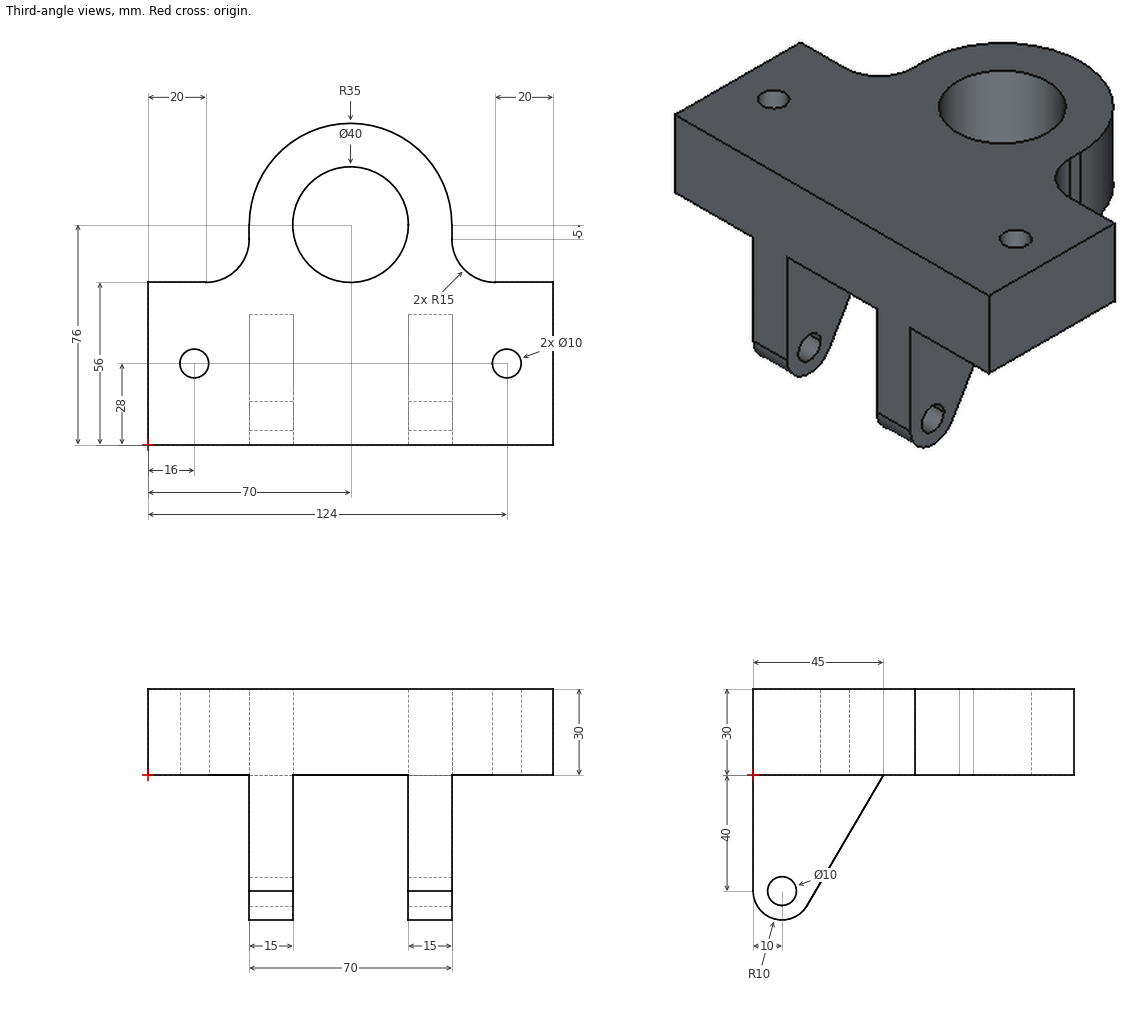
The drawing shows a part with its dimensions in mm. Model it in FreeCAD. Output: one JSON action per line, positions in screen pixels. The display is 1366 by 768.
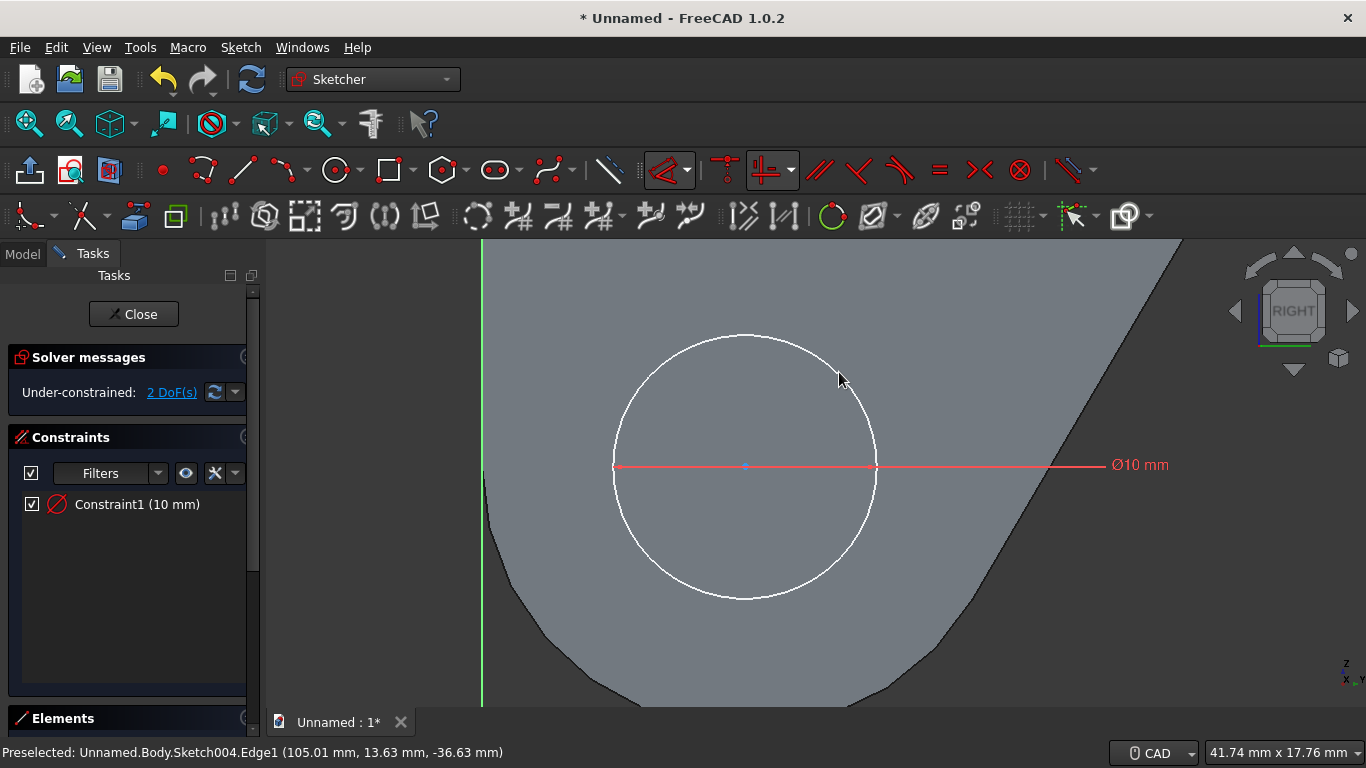
{"action": "left_click", "coordinate": [745, 467]}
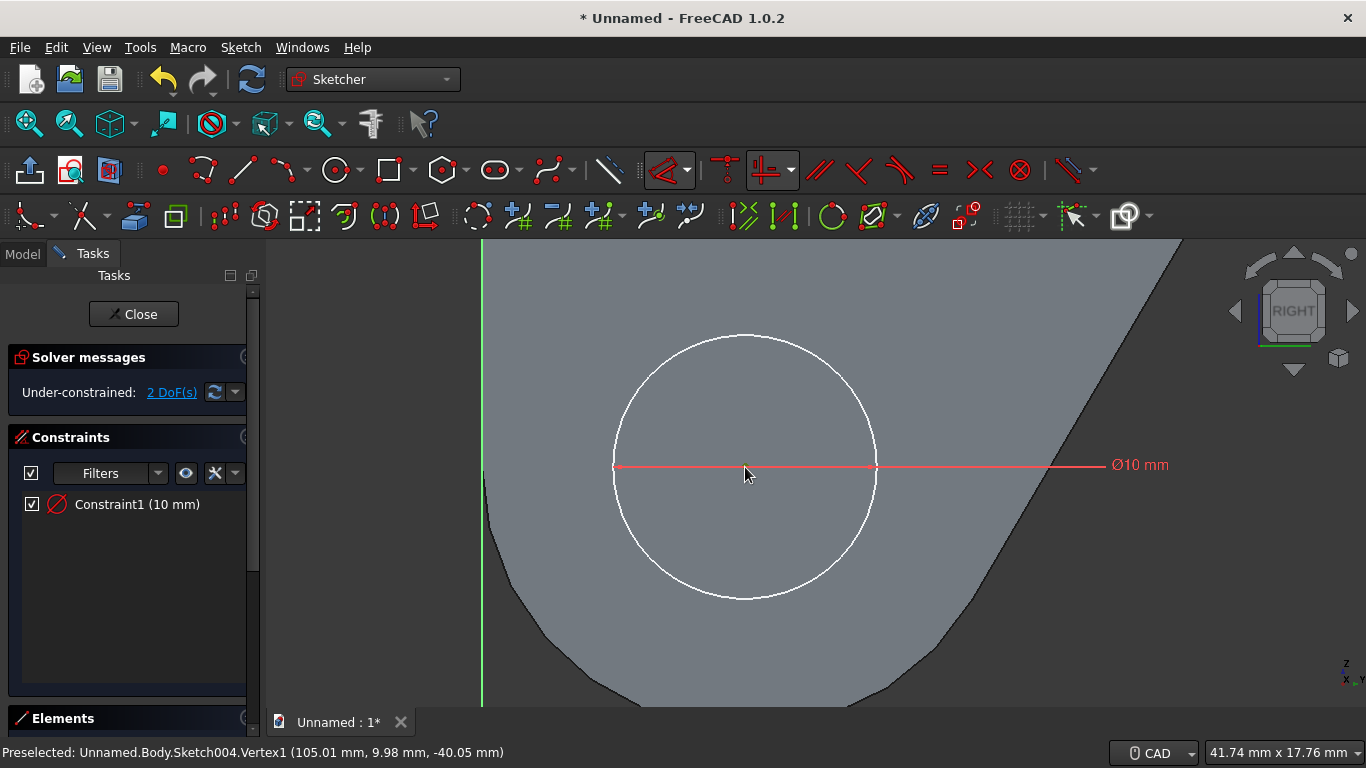
{"action": "left_click", "coordinate": [690, 170]}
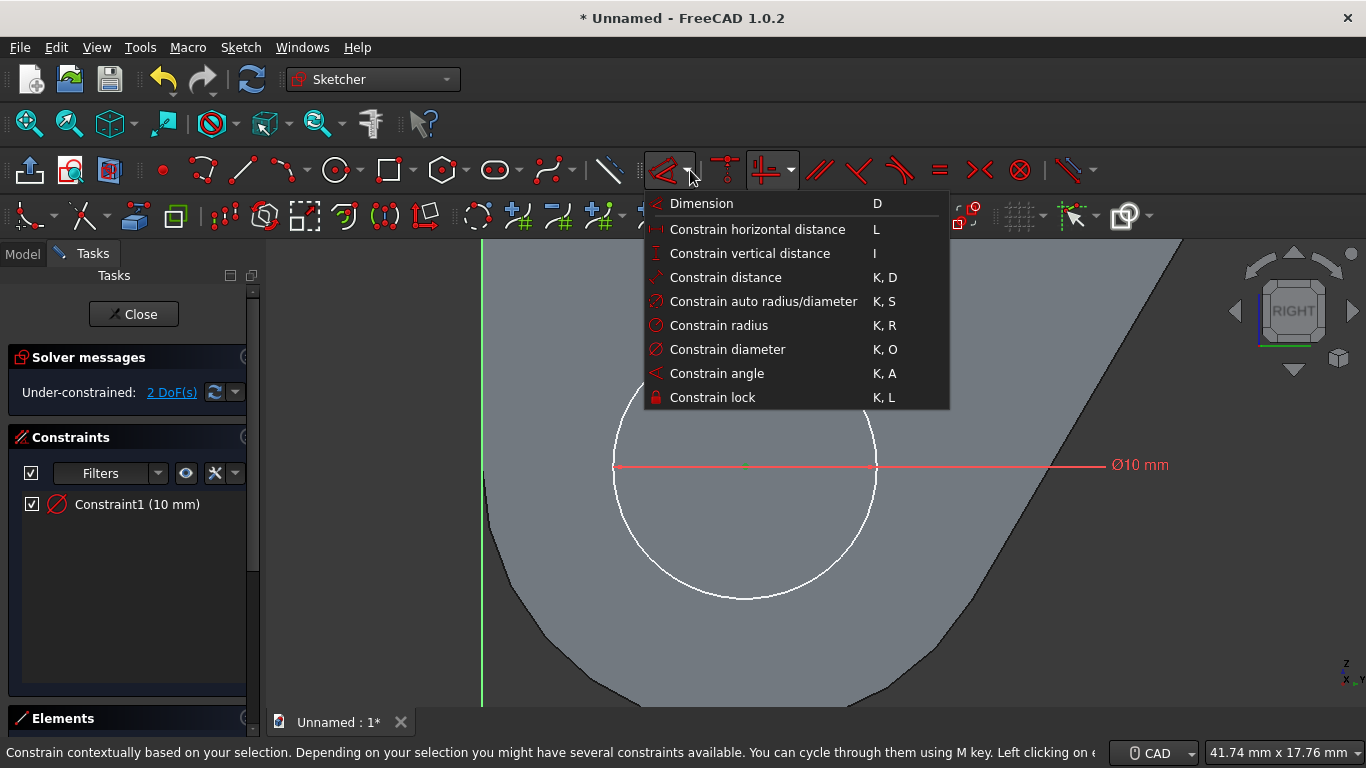
{"action": "left_click", "coordinate": [797, 229]}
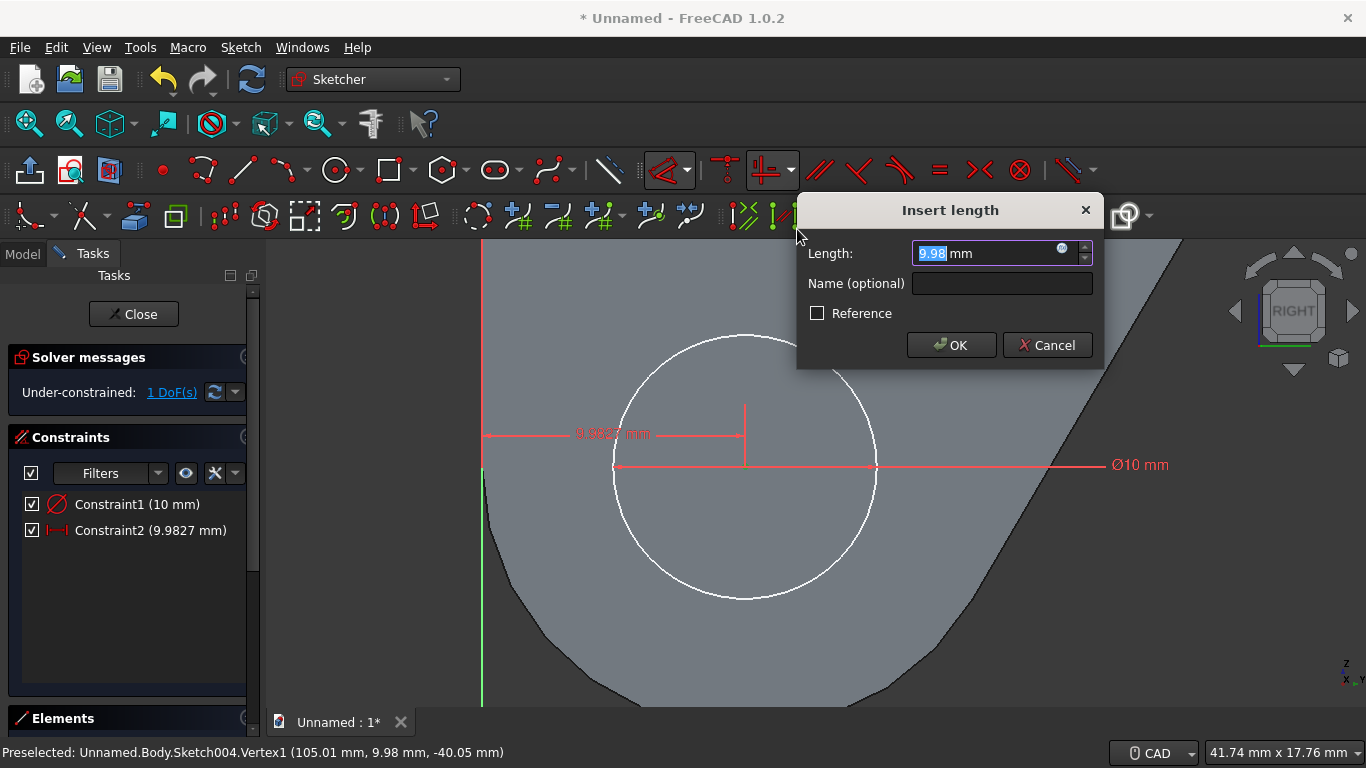
{"action": "type", "text": "10"}
{"action": "key", "text": "Return"}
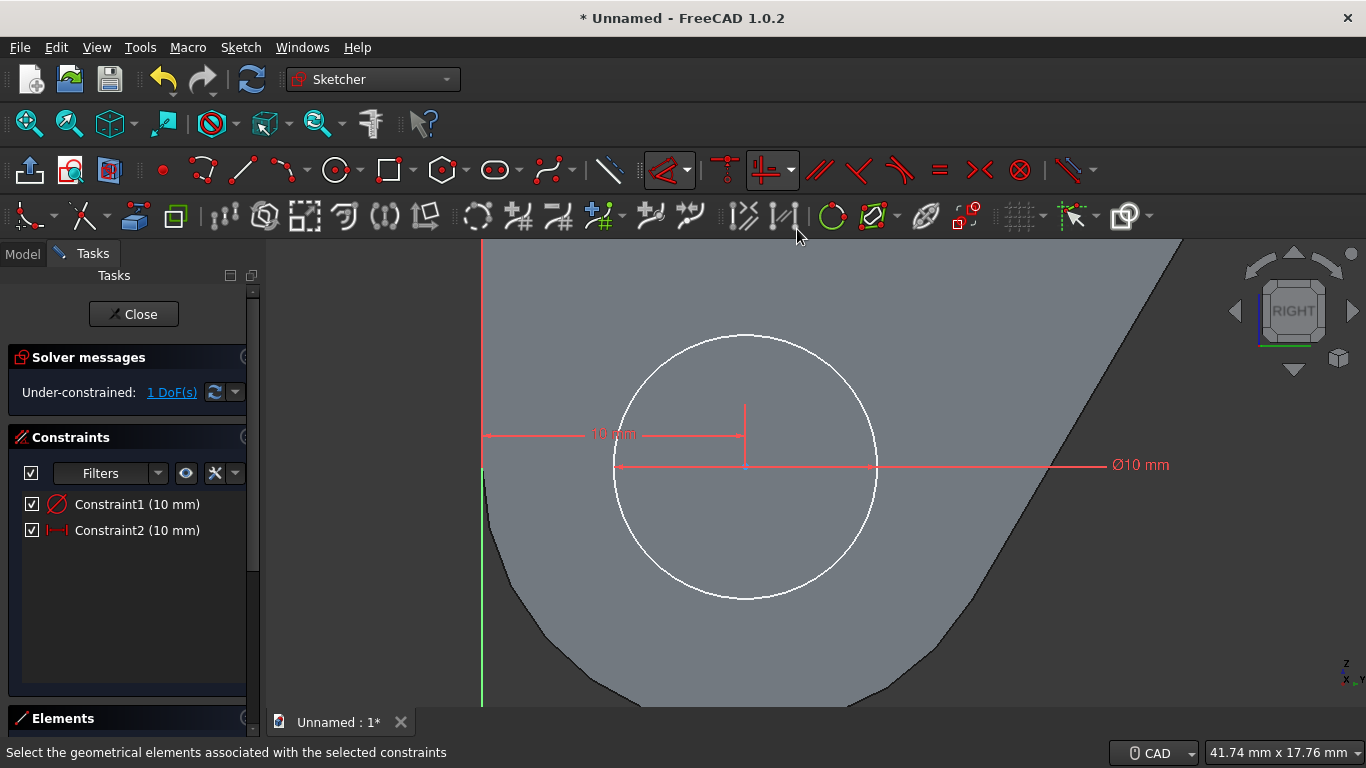
{"action": "left_click", "coordinate": [745, 467]}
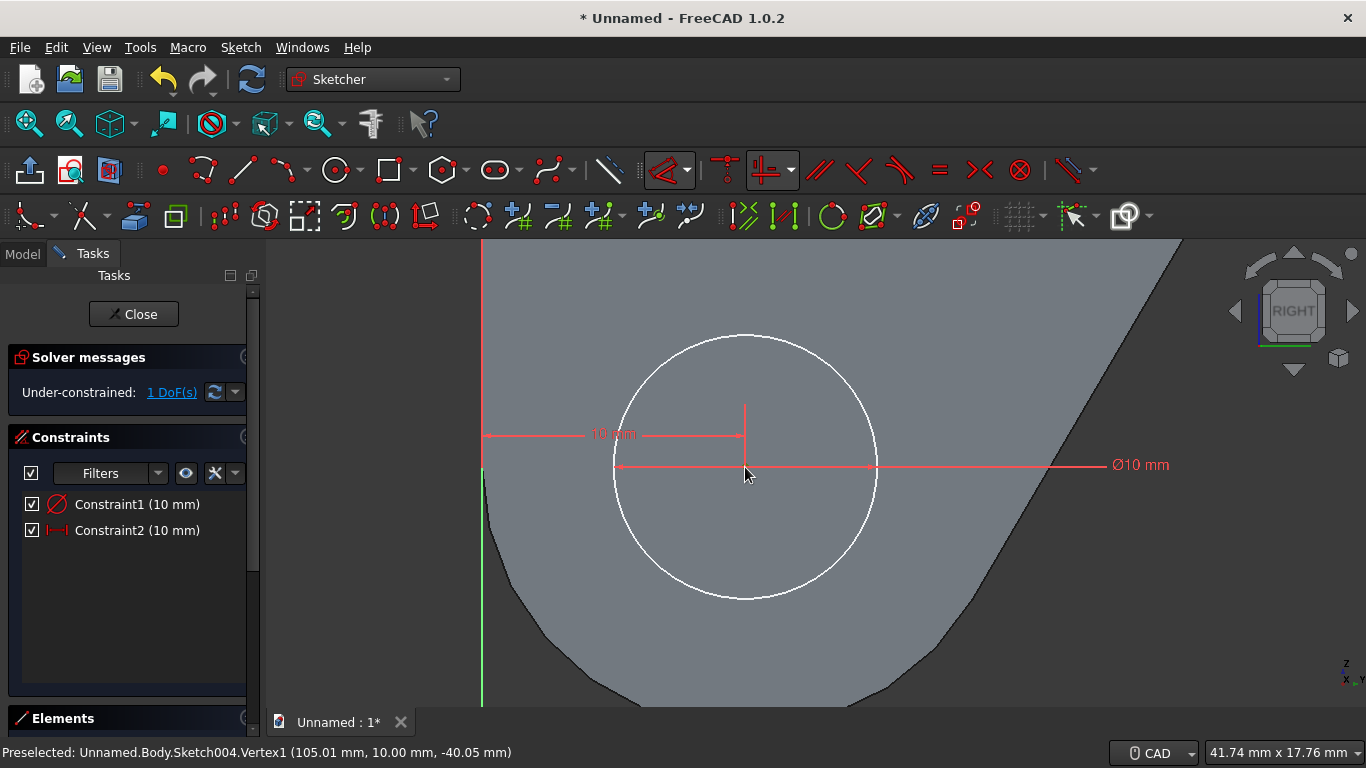
{"action": "key", "text": "i"}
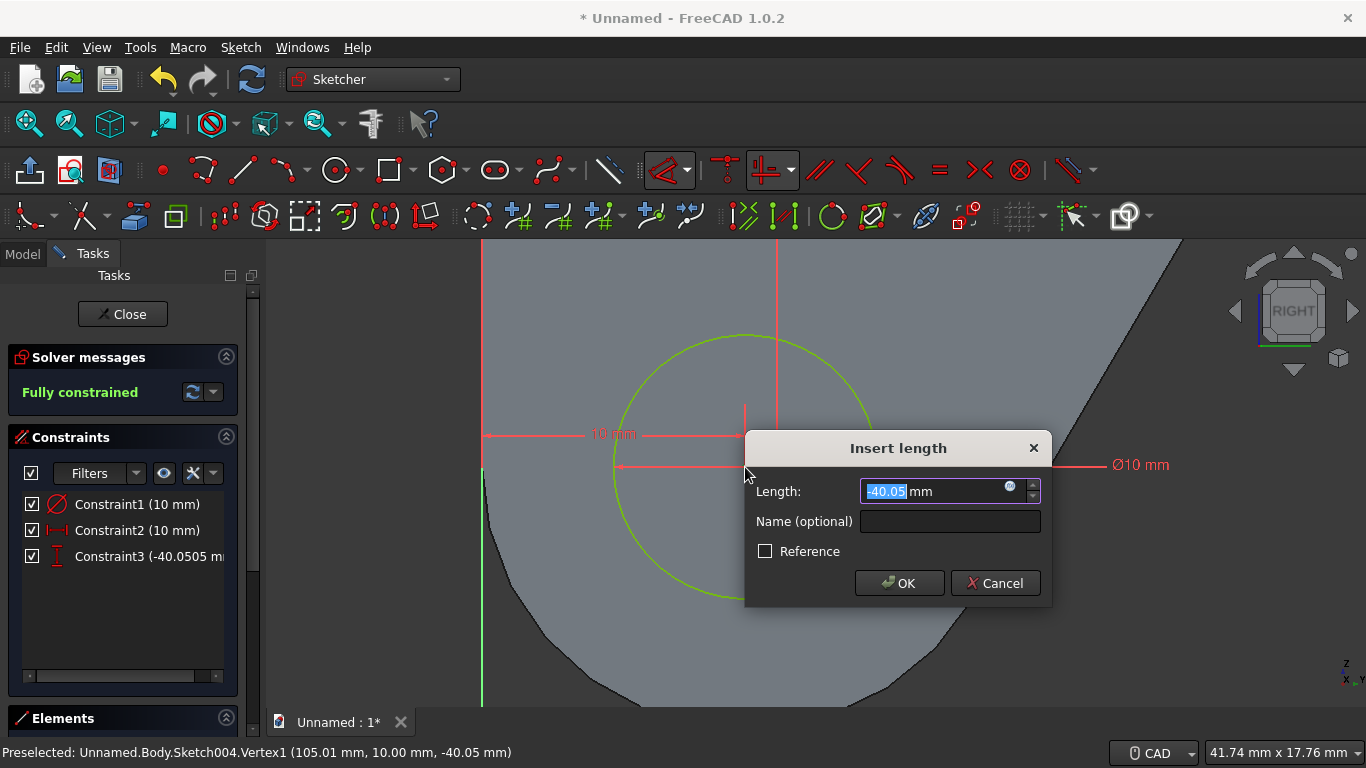
{"action": "type", "text": "-40"}
{"action": "key", "text": "Return"}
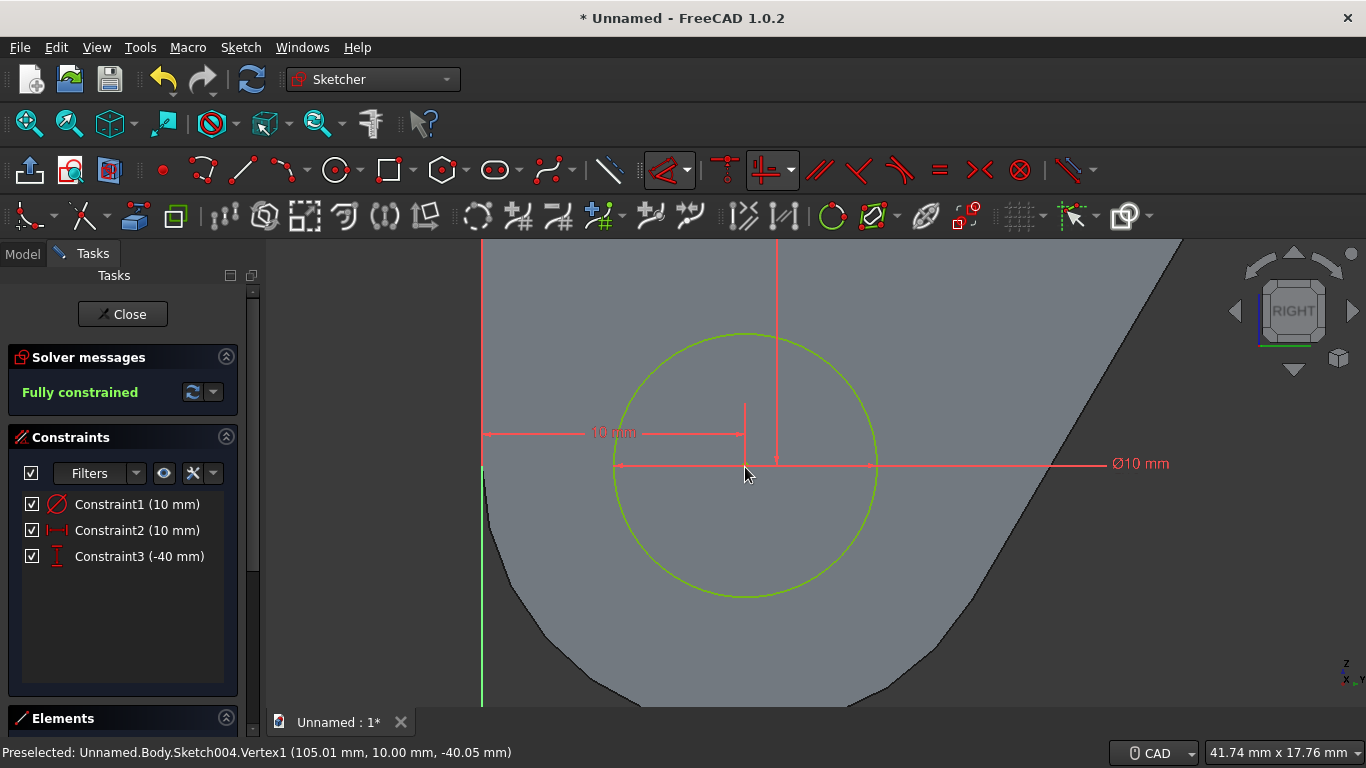
{"action": "left_click", "coordinate": [123, 314]}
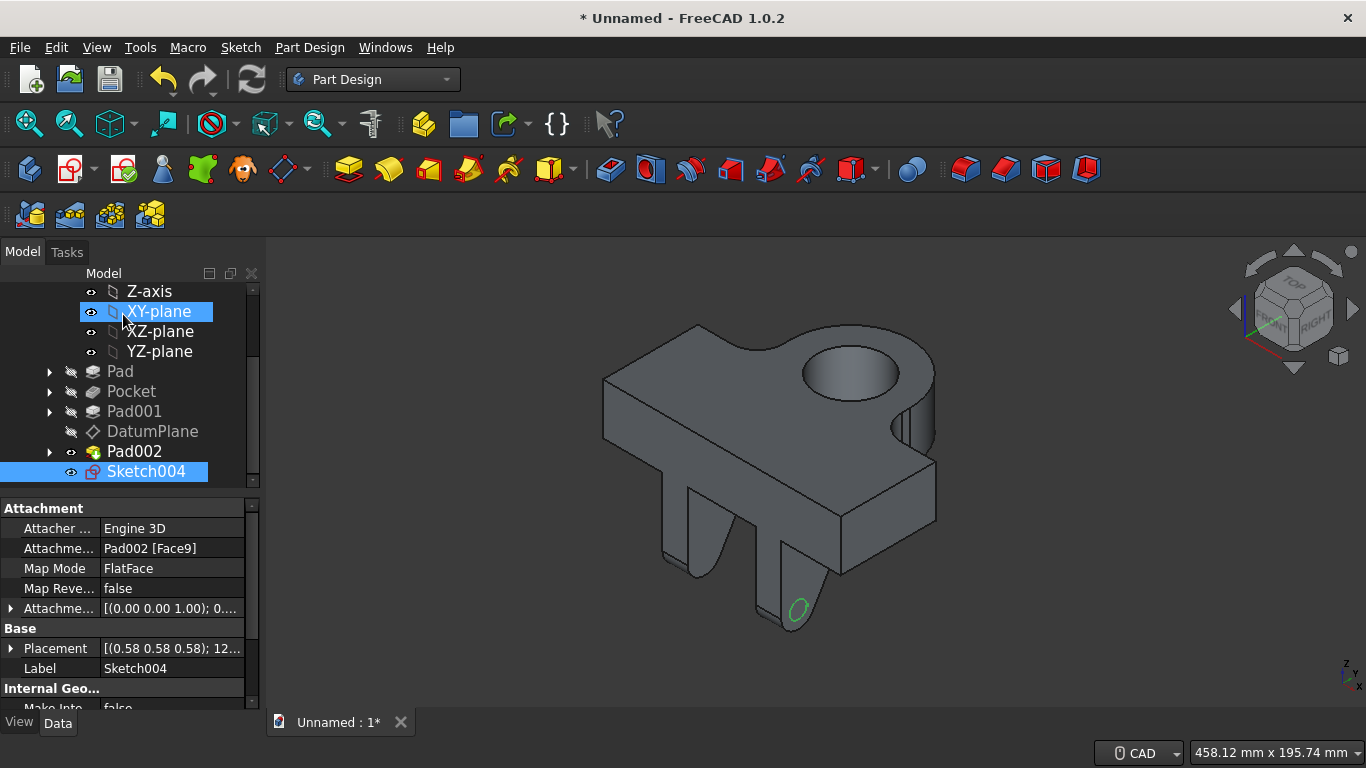
{"action": "left_click", "coordinate": [612, 170]}